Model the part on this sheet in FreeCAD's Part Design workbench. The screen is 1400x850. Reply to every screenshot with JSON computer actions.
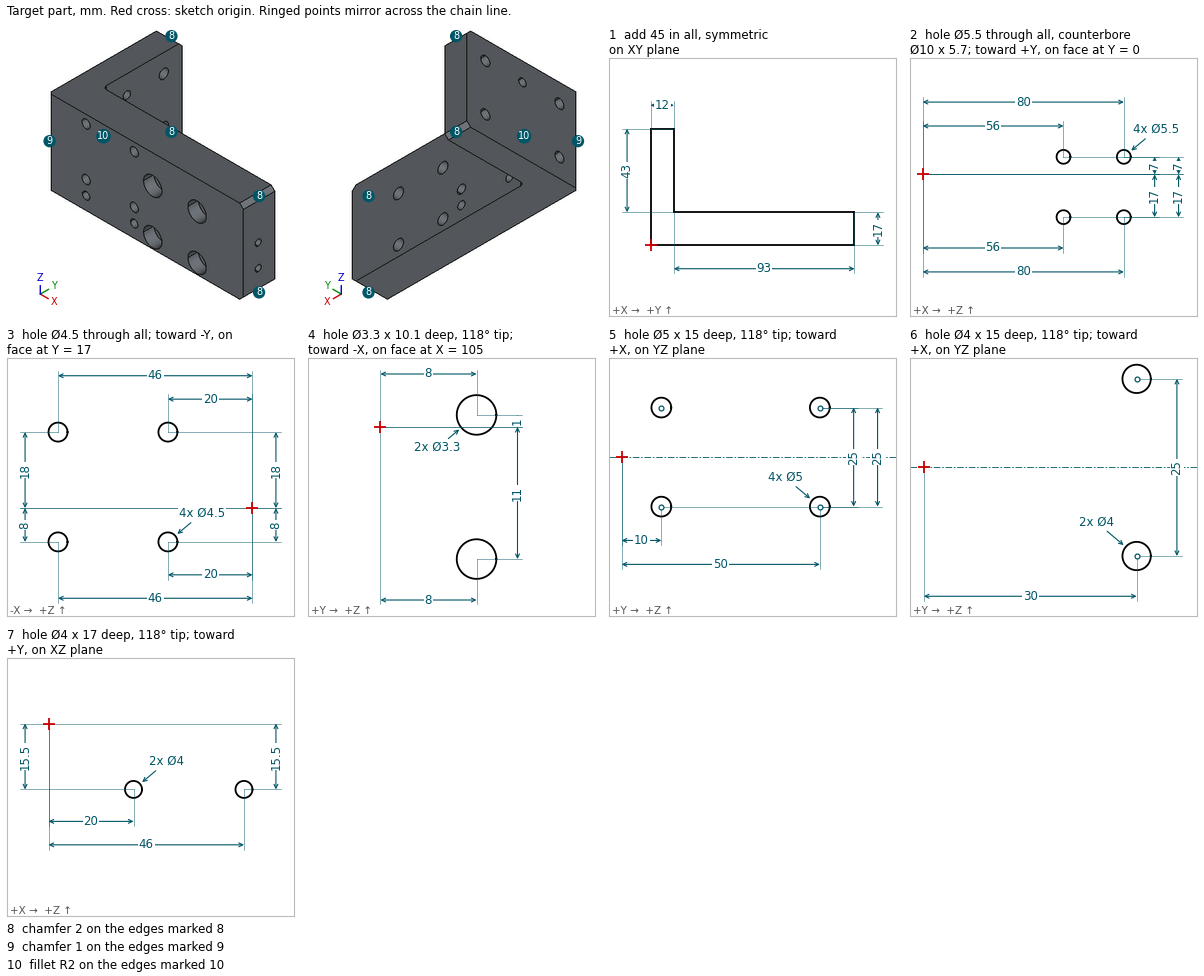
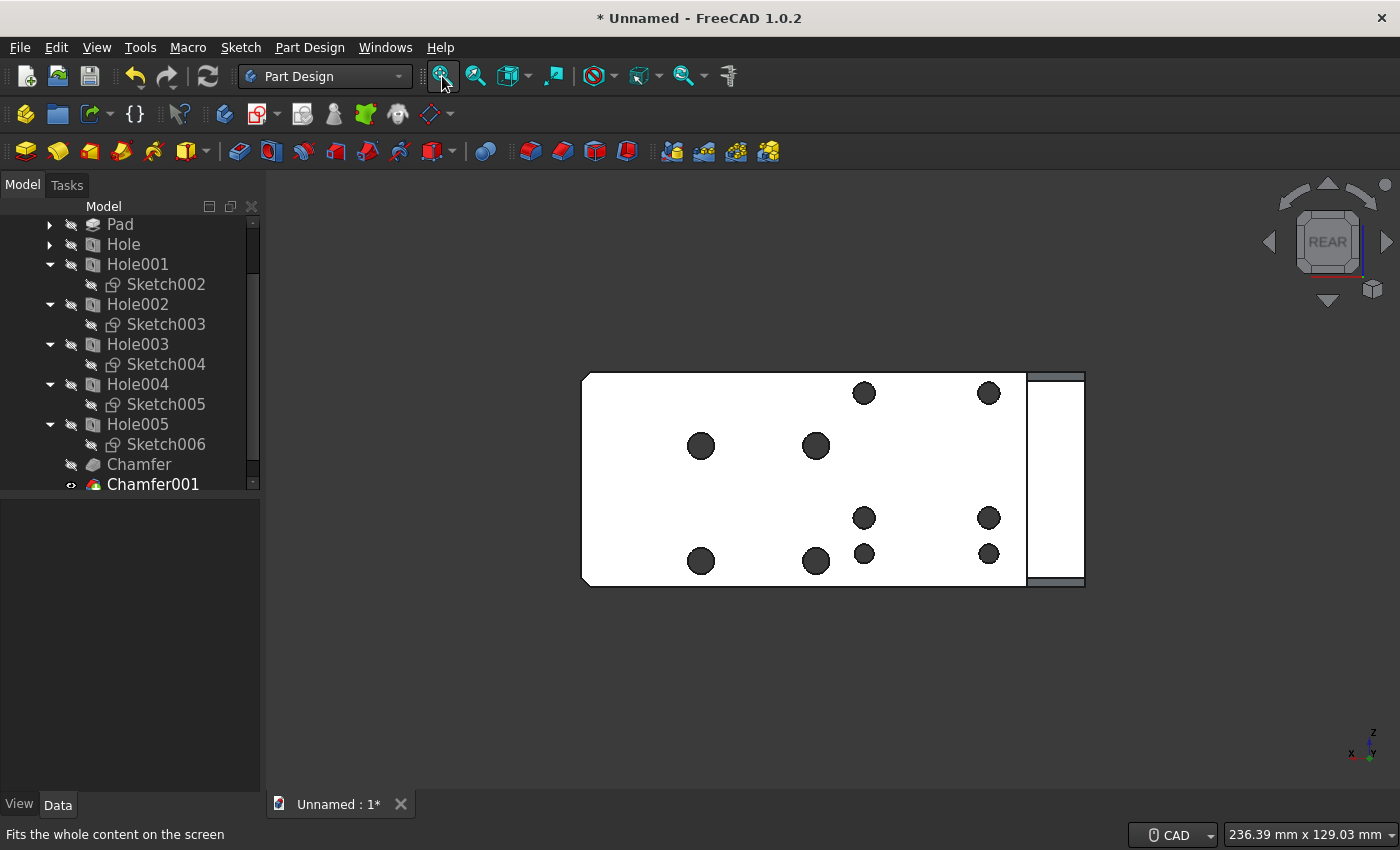
{"action": "key", "text": "v f"}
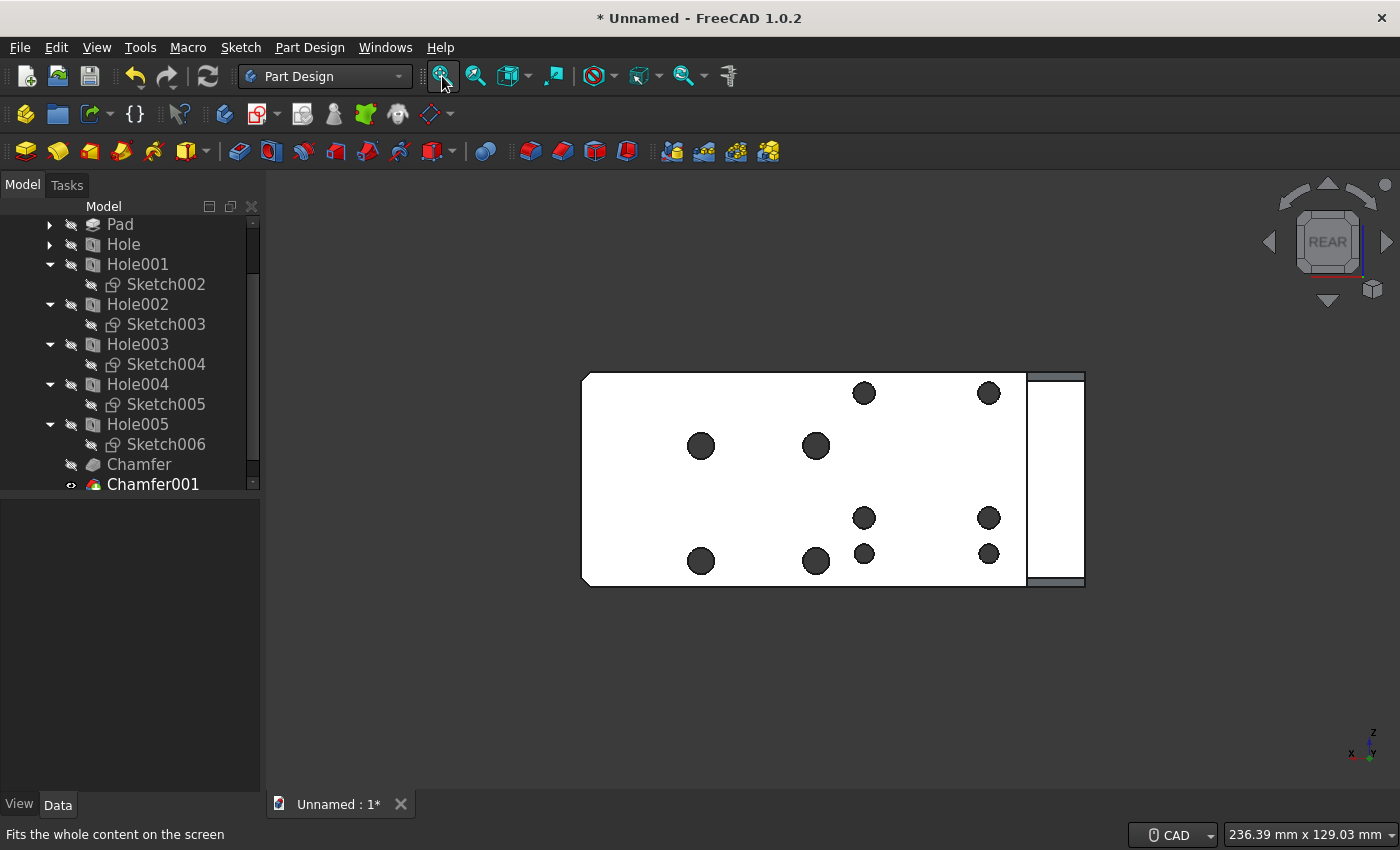
{"action": "key", "text": "6"}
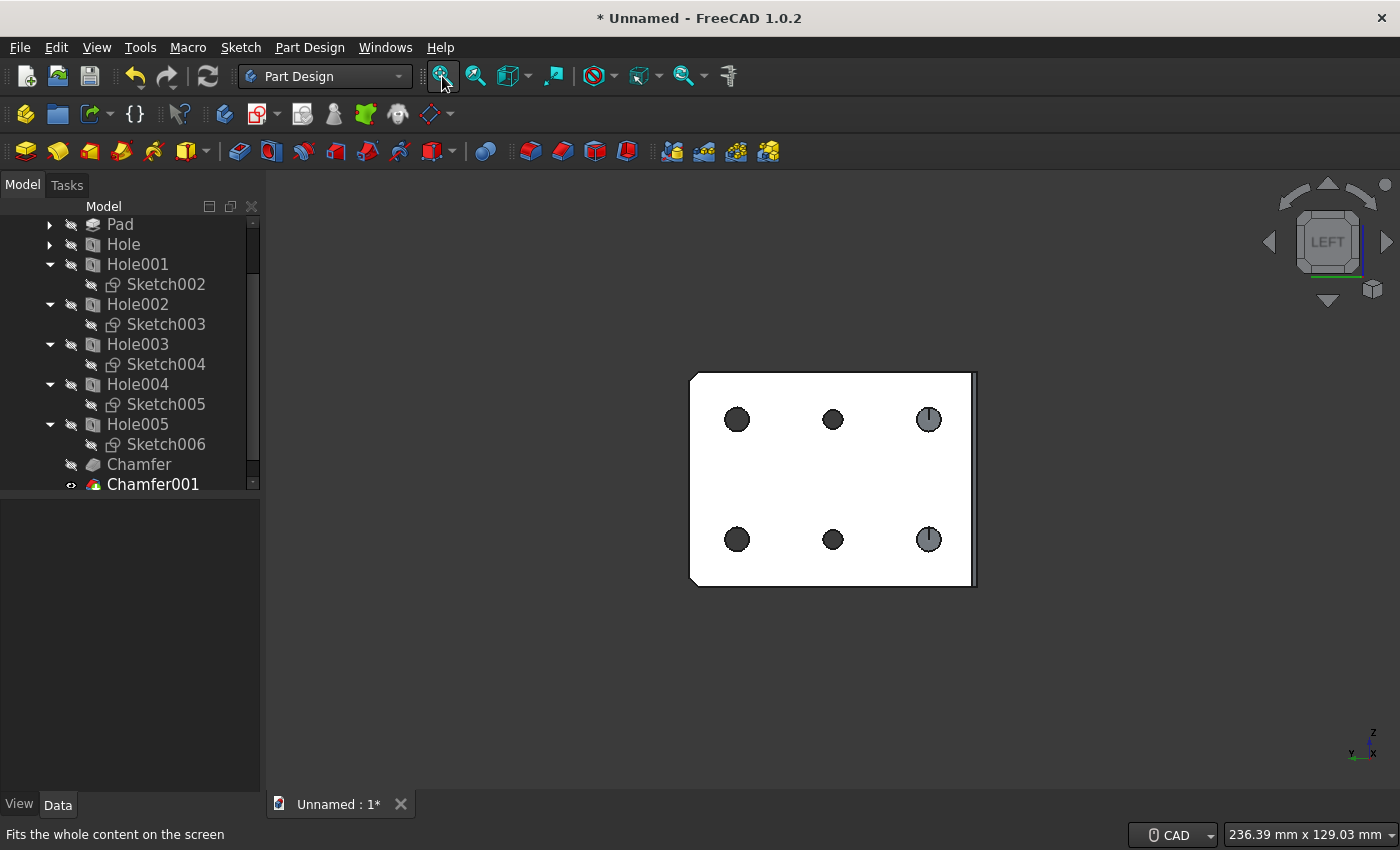
{"action": "key", "text": "v f"}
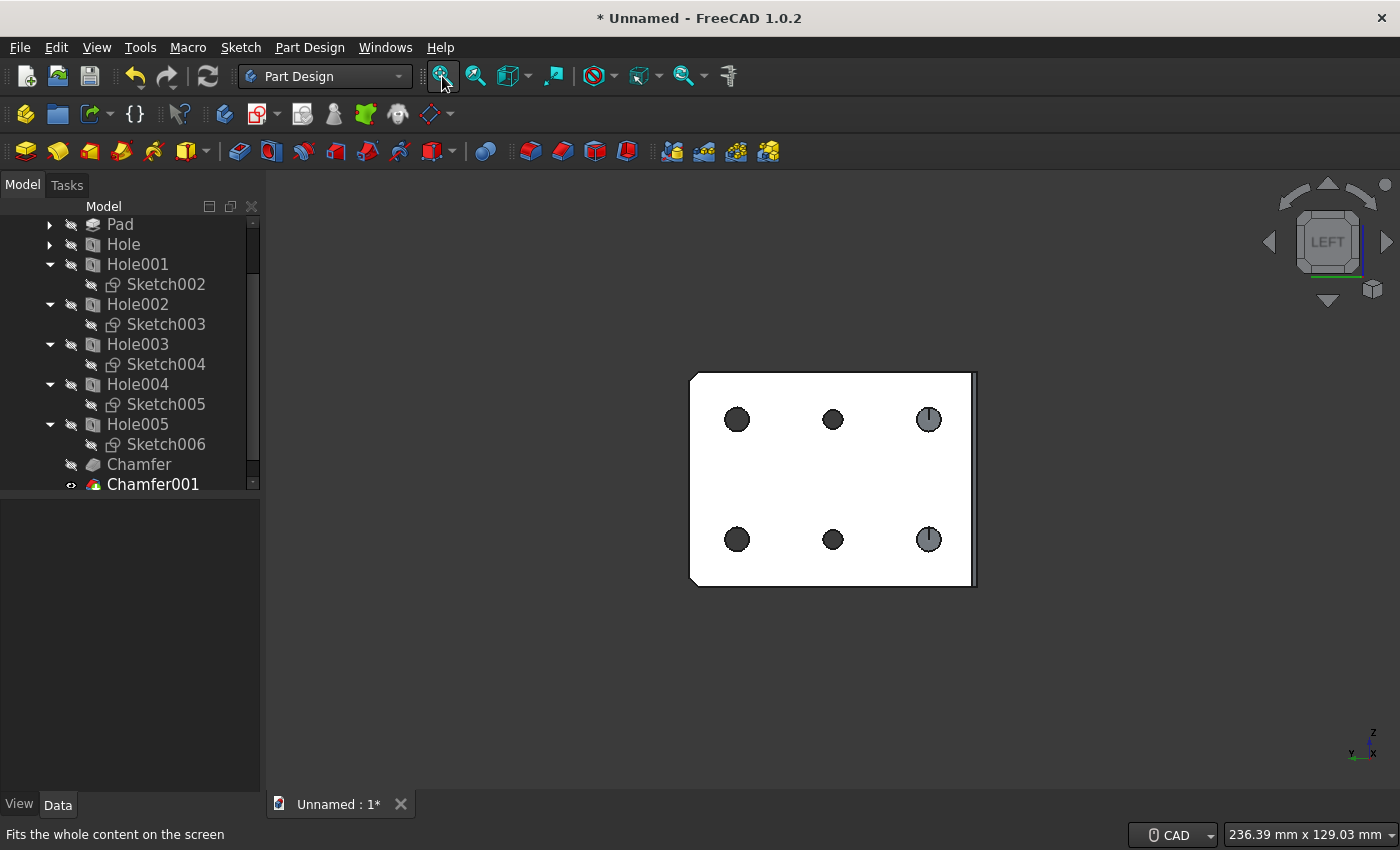
{"action": "key", "text": "v 3"}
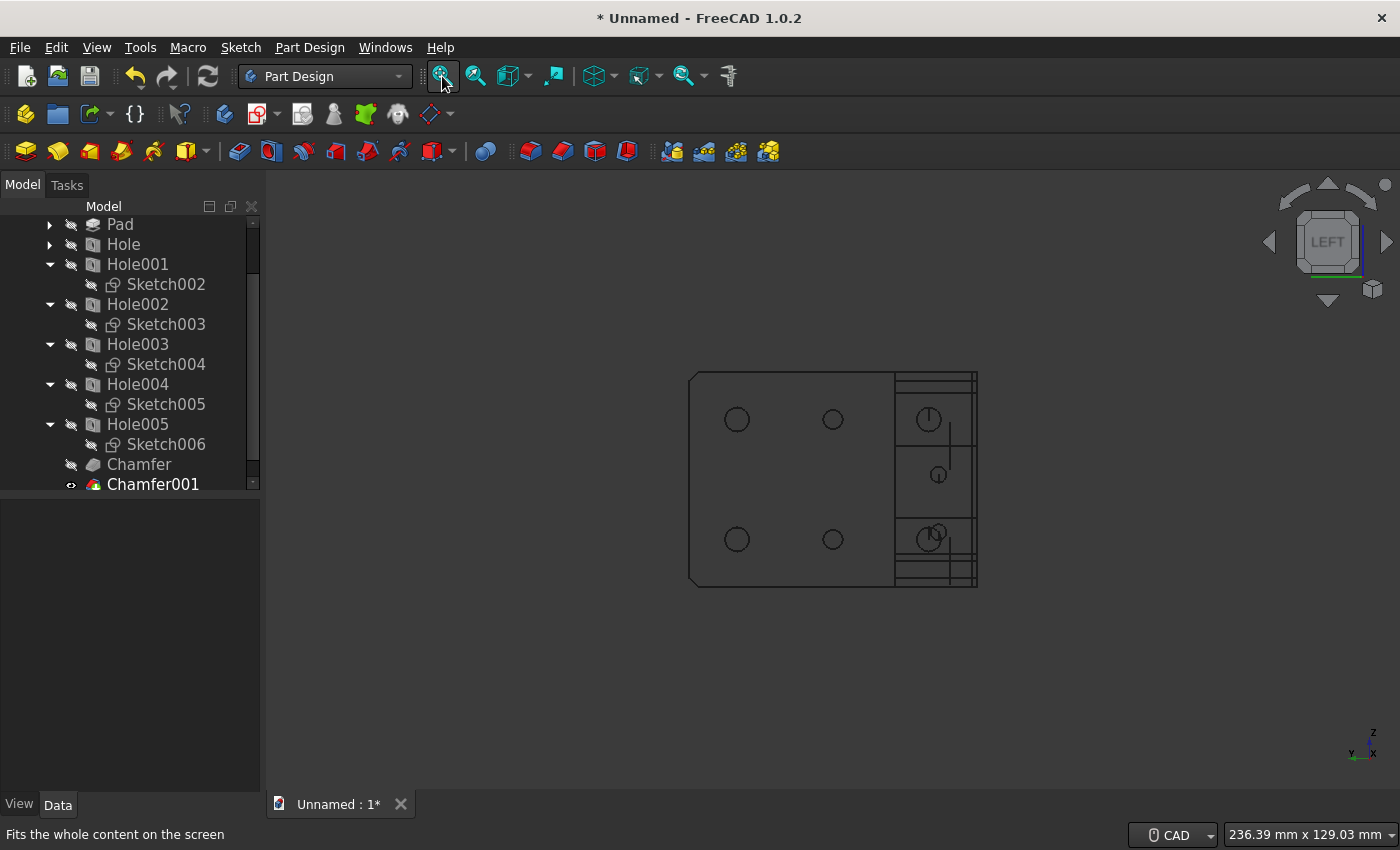
{"action": "key", "text": "0"}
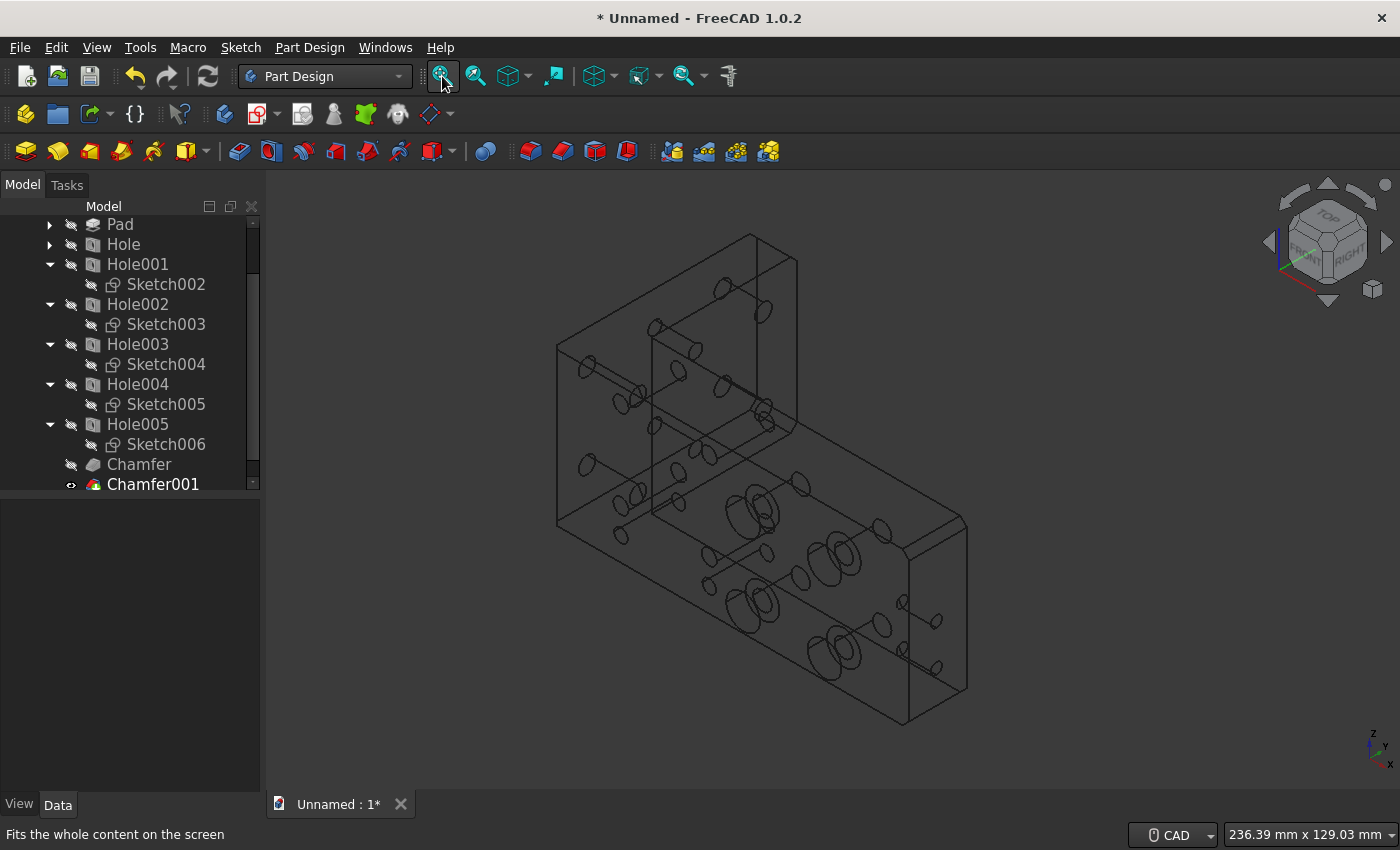
{"action": "left_click", "coordinate": [652, 425]}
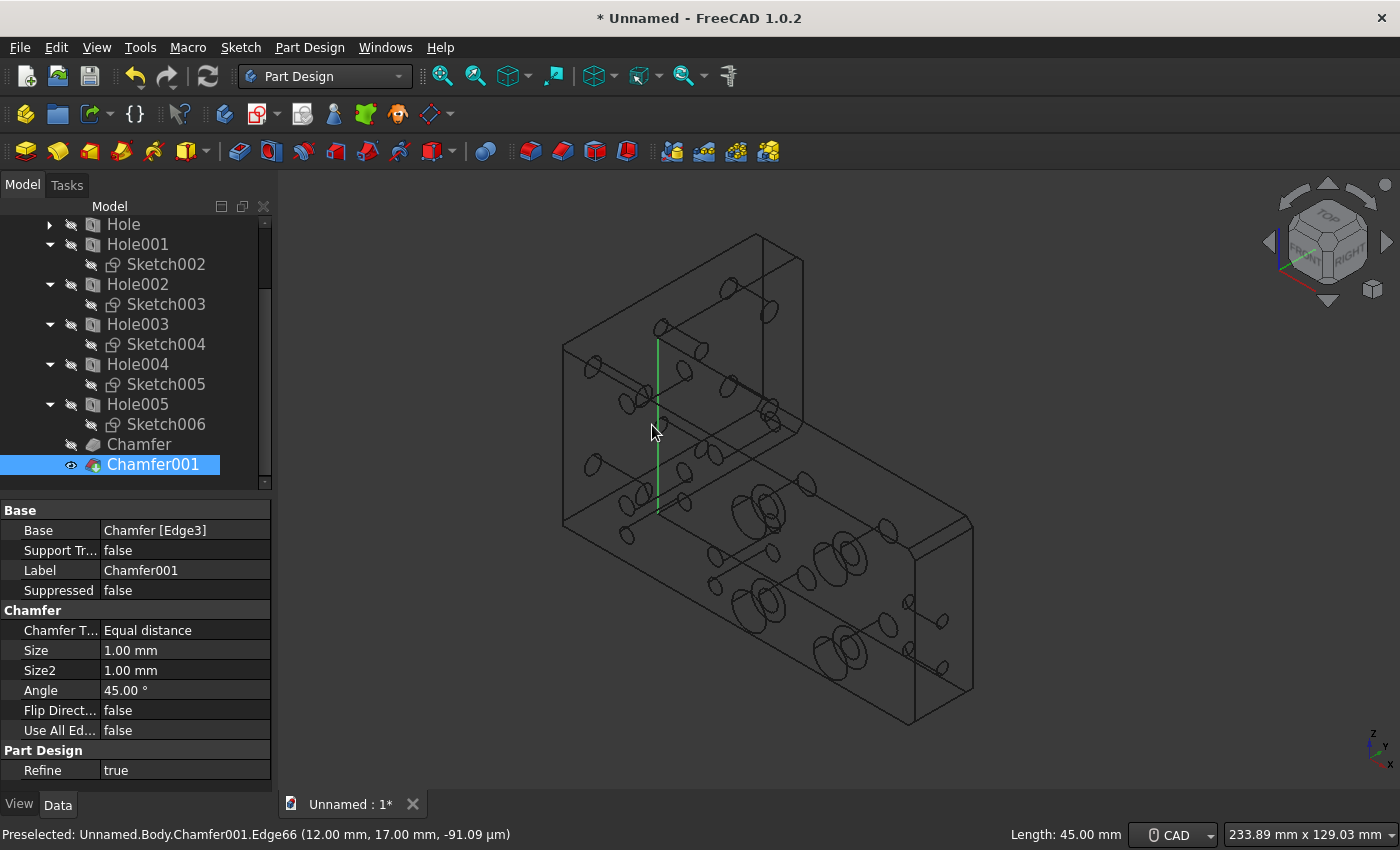
{"action": "key", "text": "v 1"}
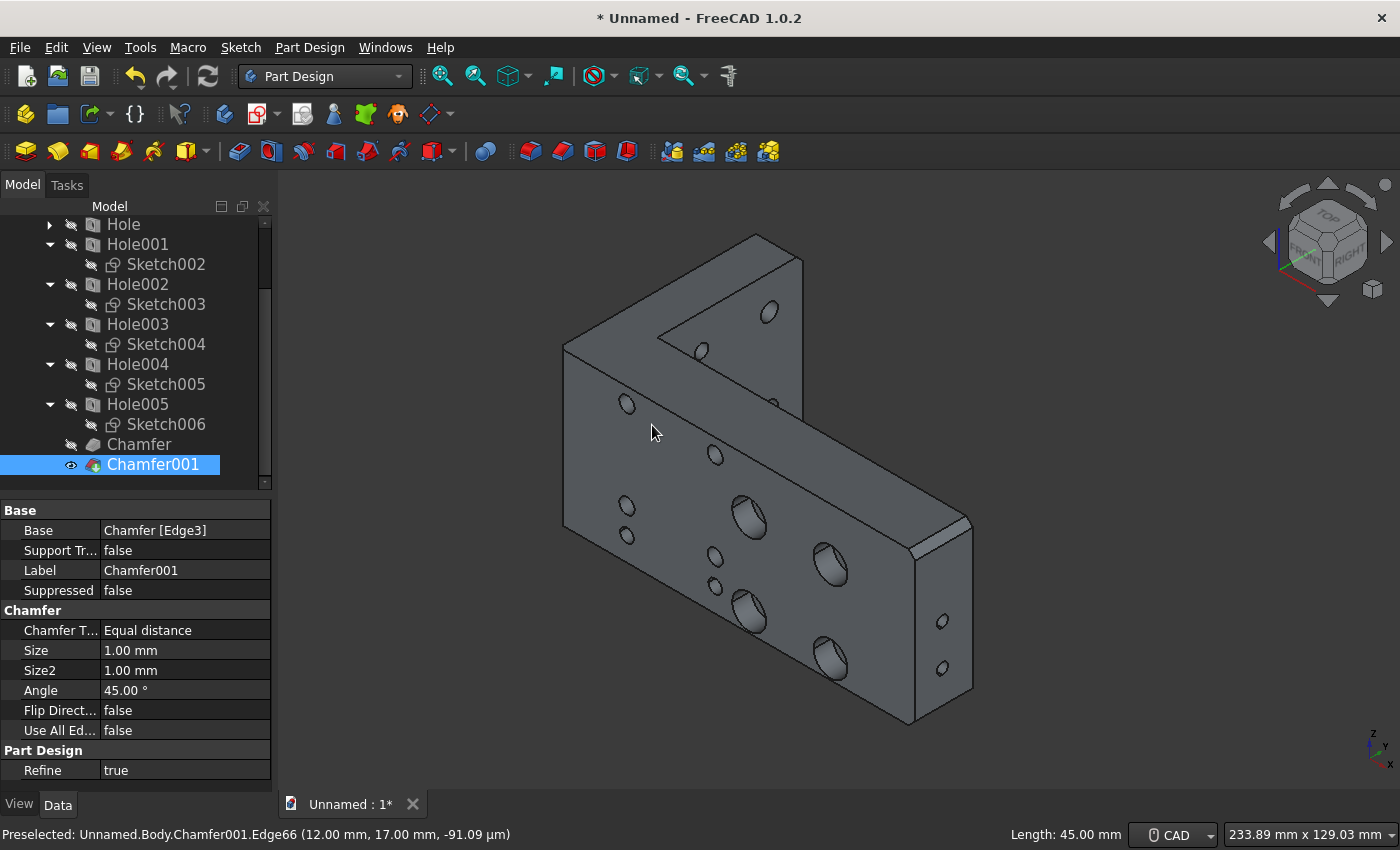
{"action": "left_click", "coordinate": [532, 152]}